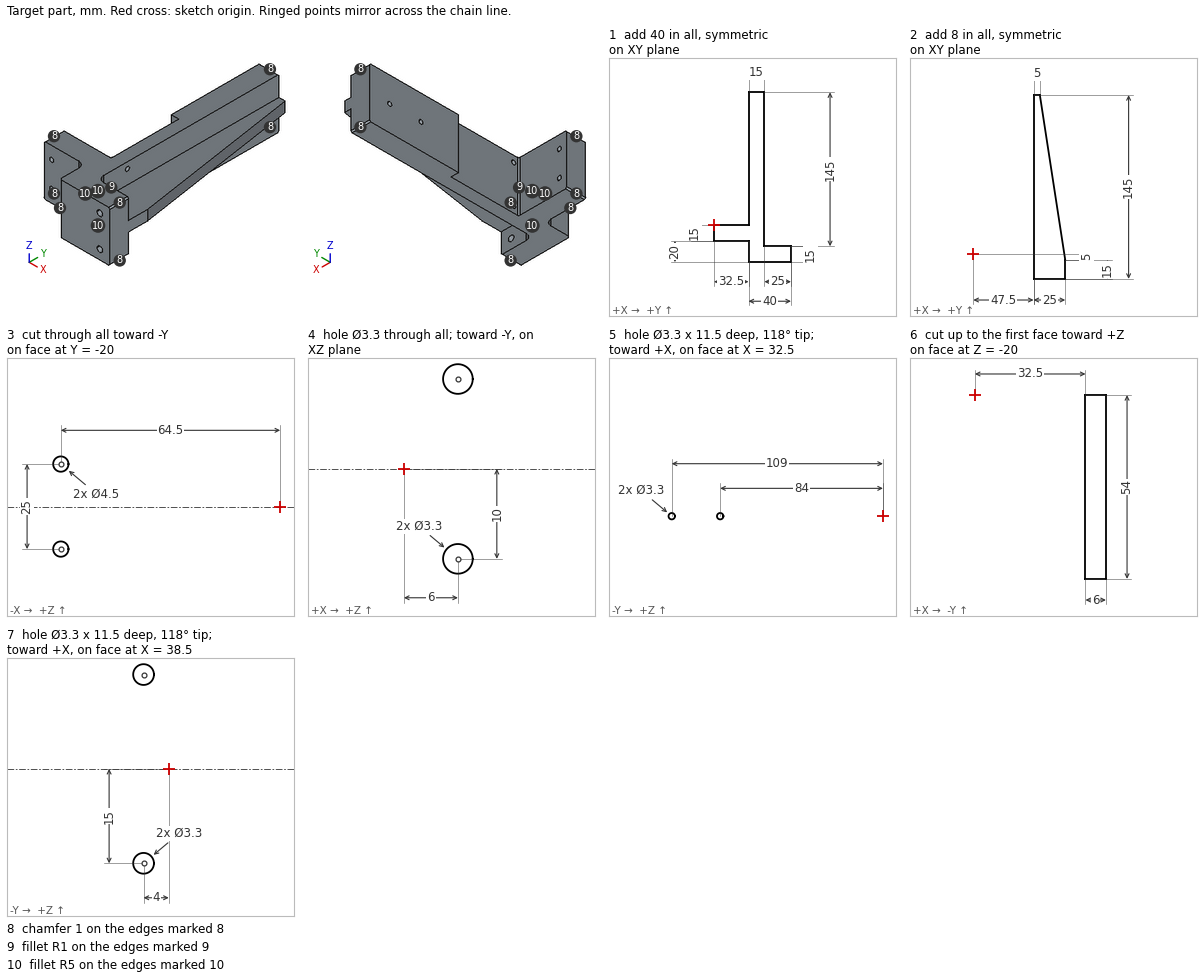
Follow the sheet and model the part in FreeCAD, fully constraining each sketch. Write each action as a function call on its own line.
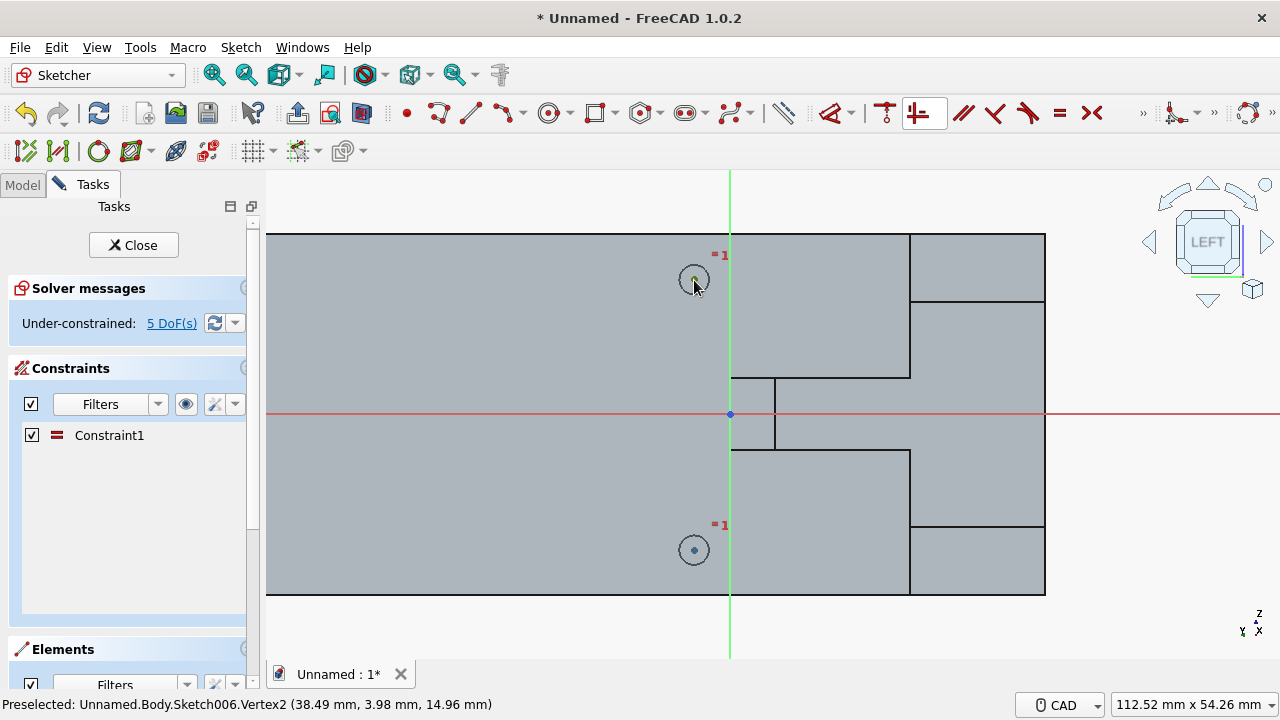
click(353, 414)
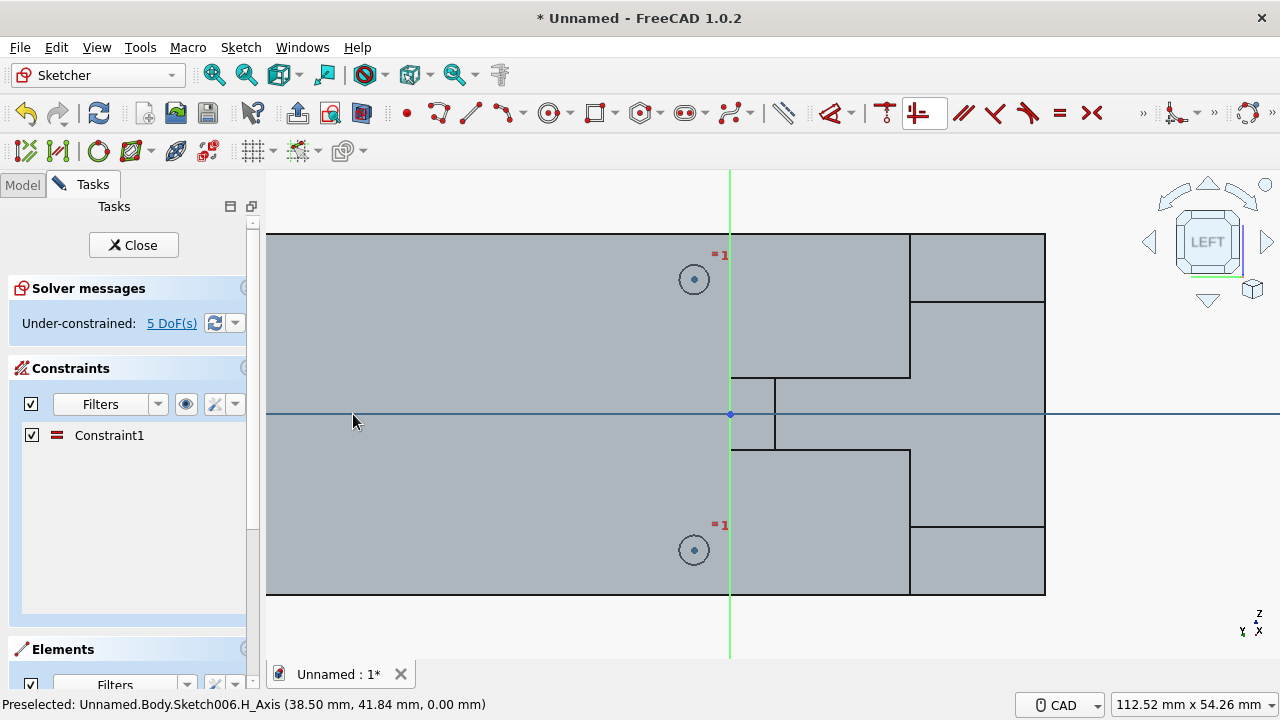
click(1092, 114)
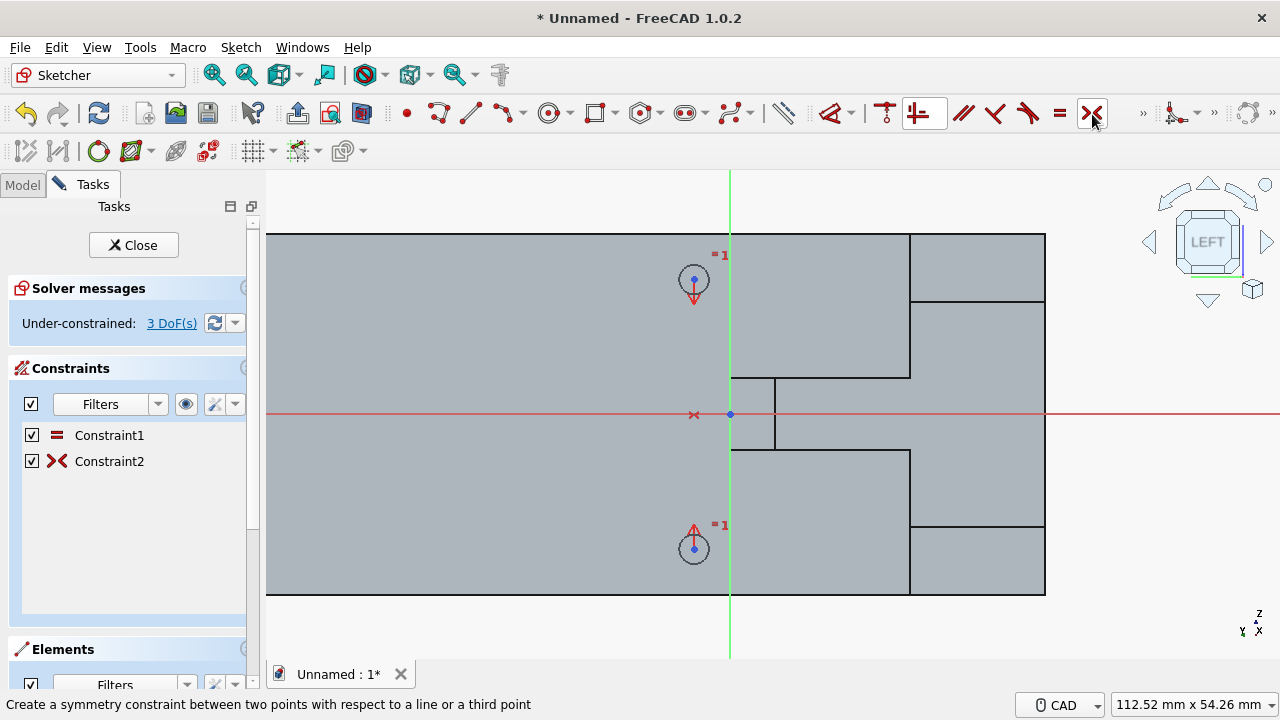
key(d)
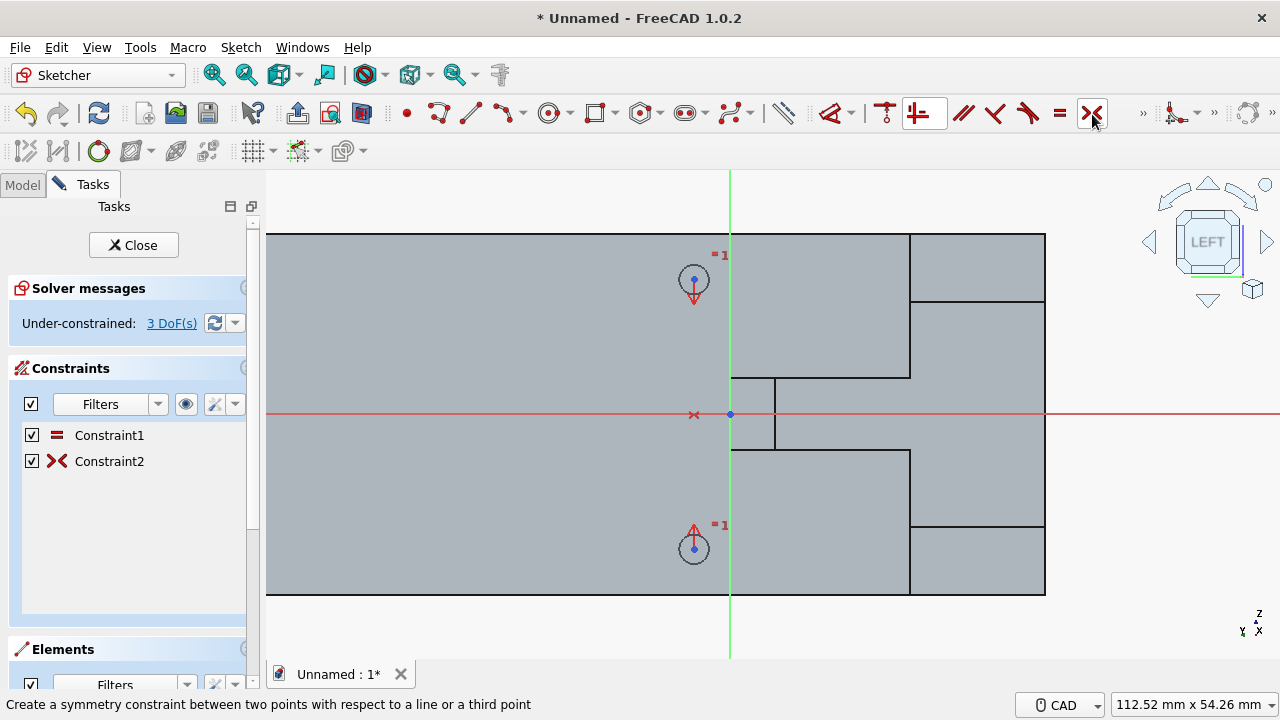
scroll(704, 539, up, 2)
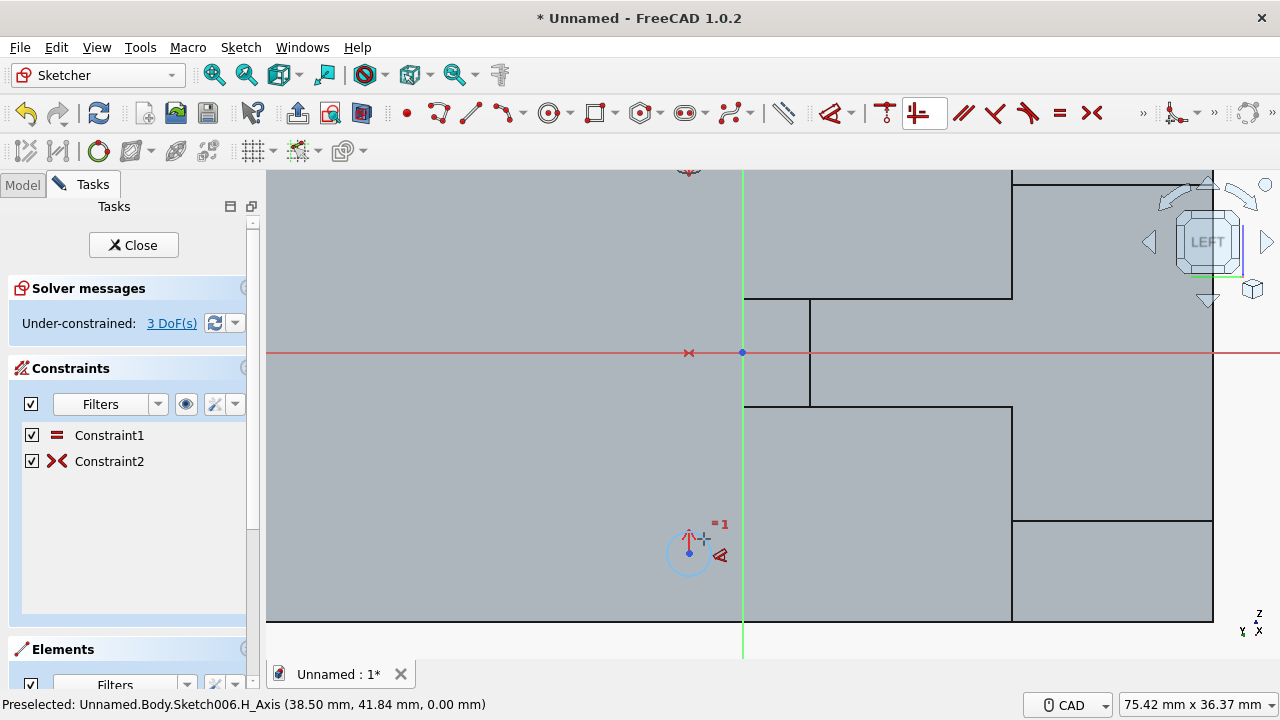
click(705, 538)
click(728, 515)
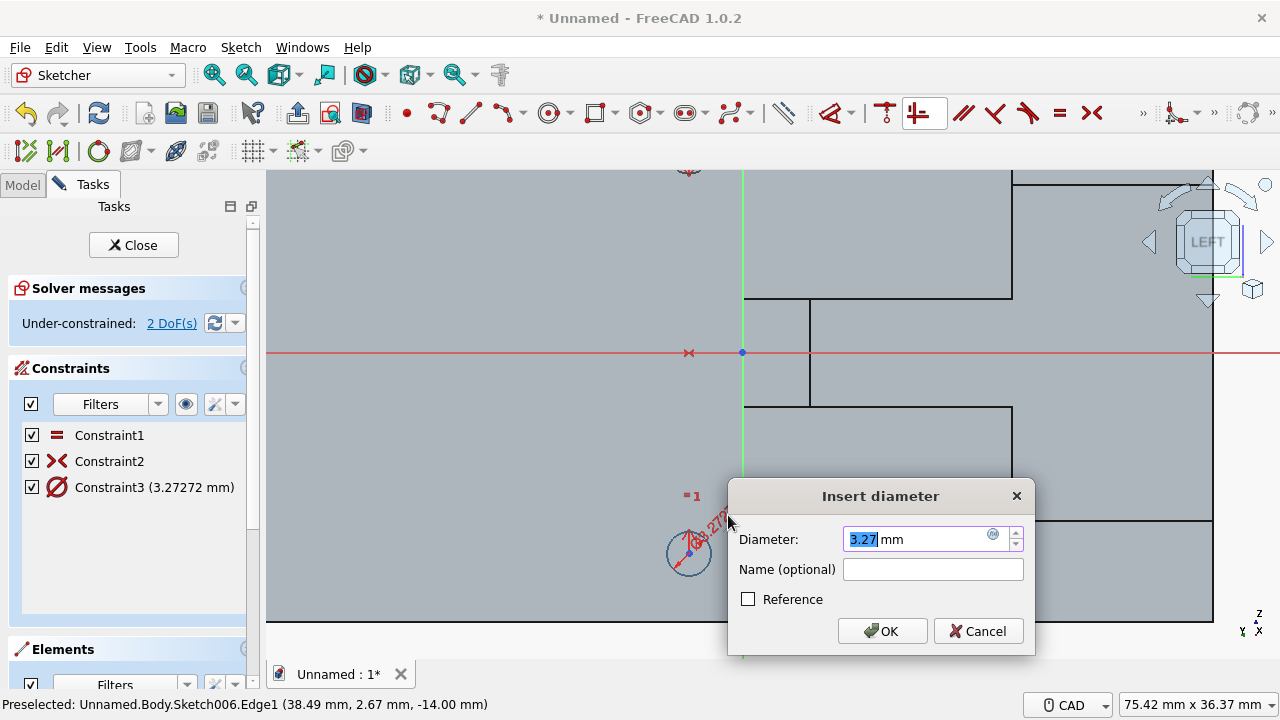
text(3.3)
key(Return)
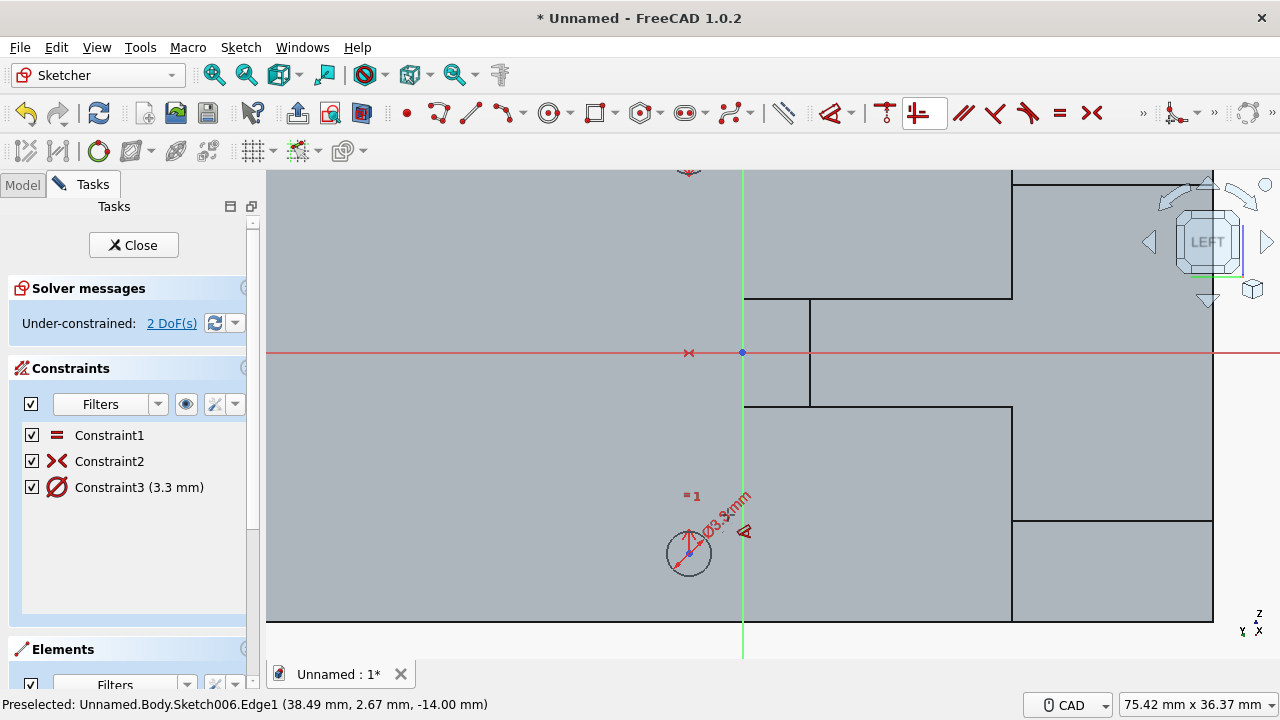
click(689, 554)
click(716, 588)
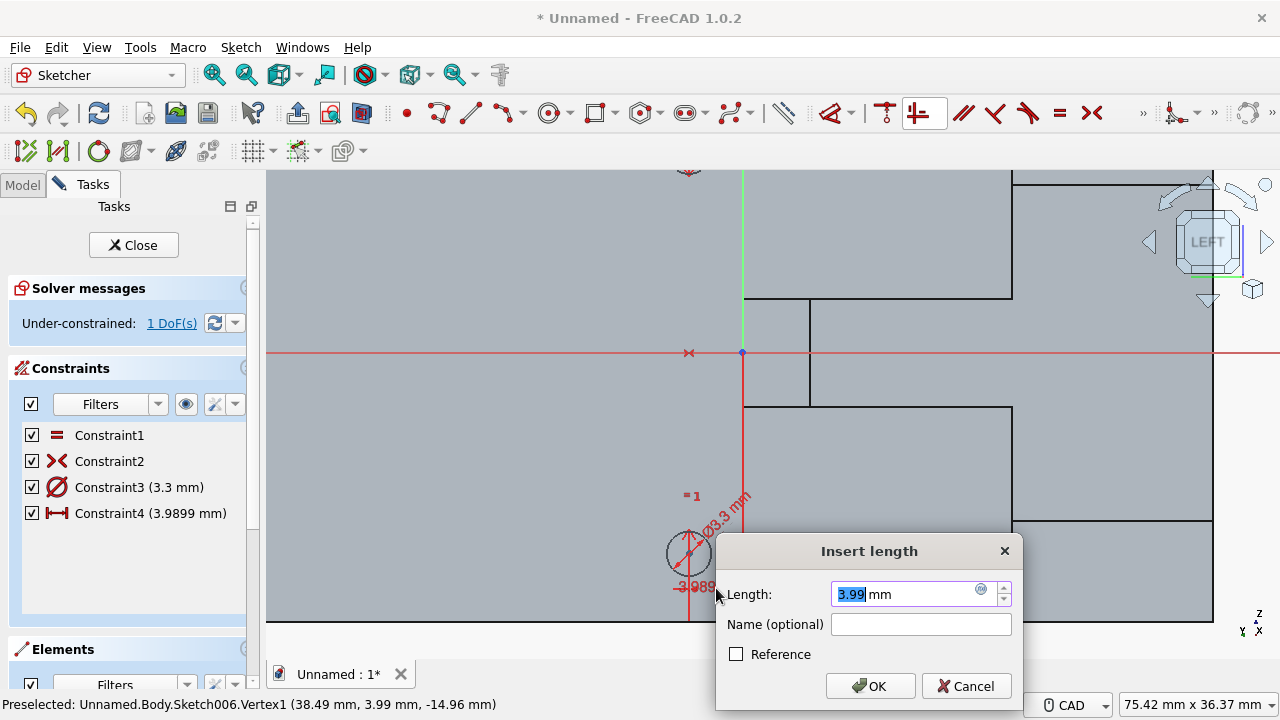
text(4)
key(Return)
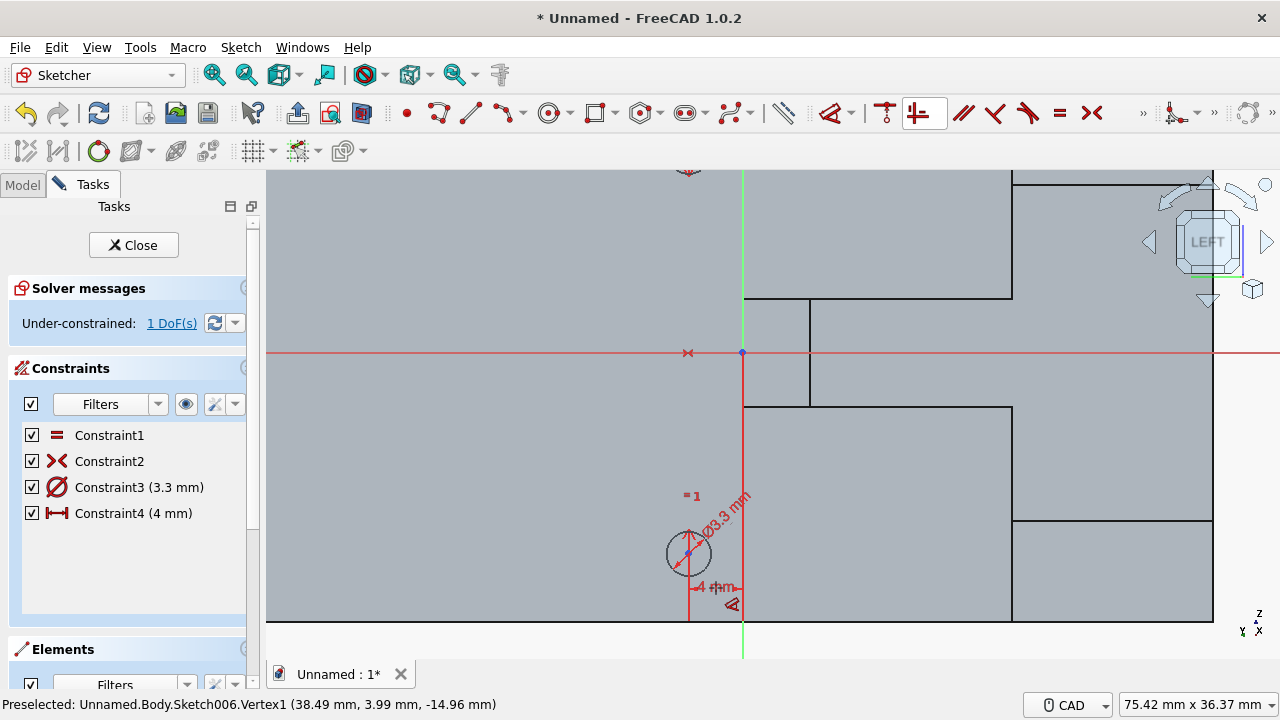
click(689, 554)
click(777, 453)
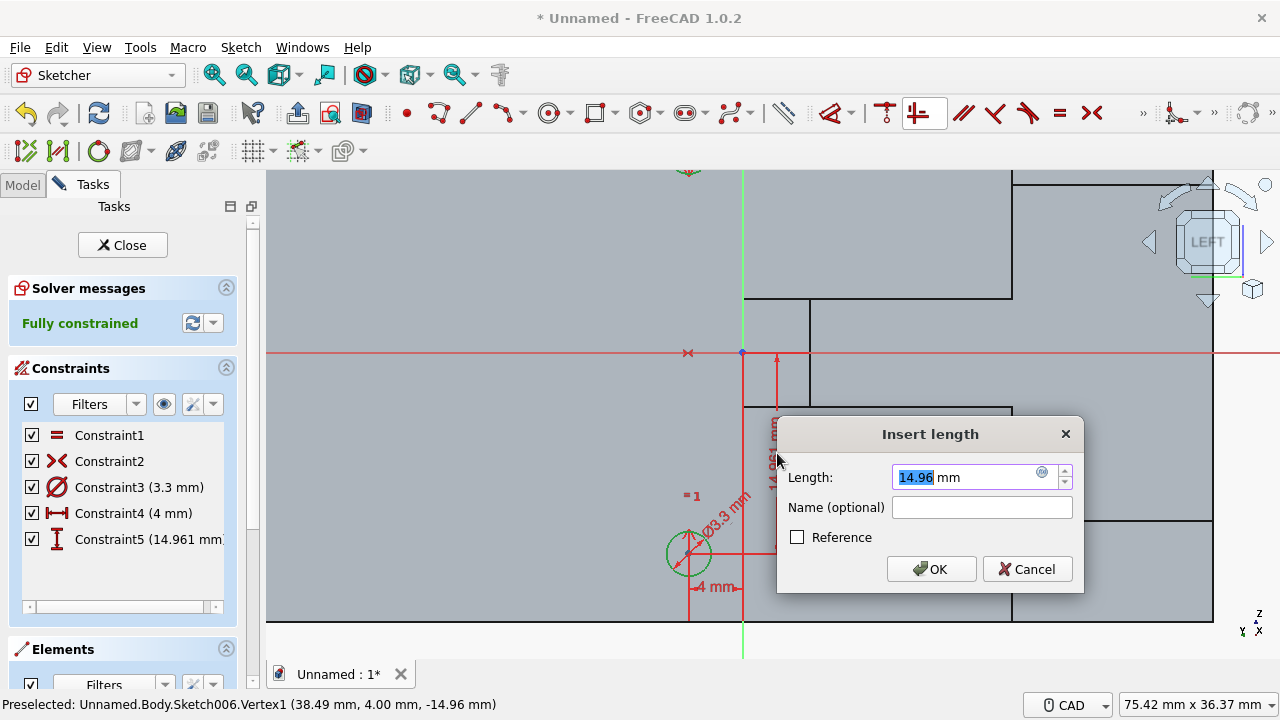
text(15)
key(Return)
key(Escape)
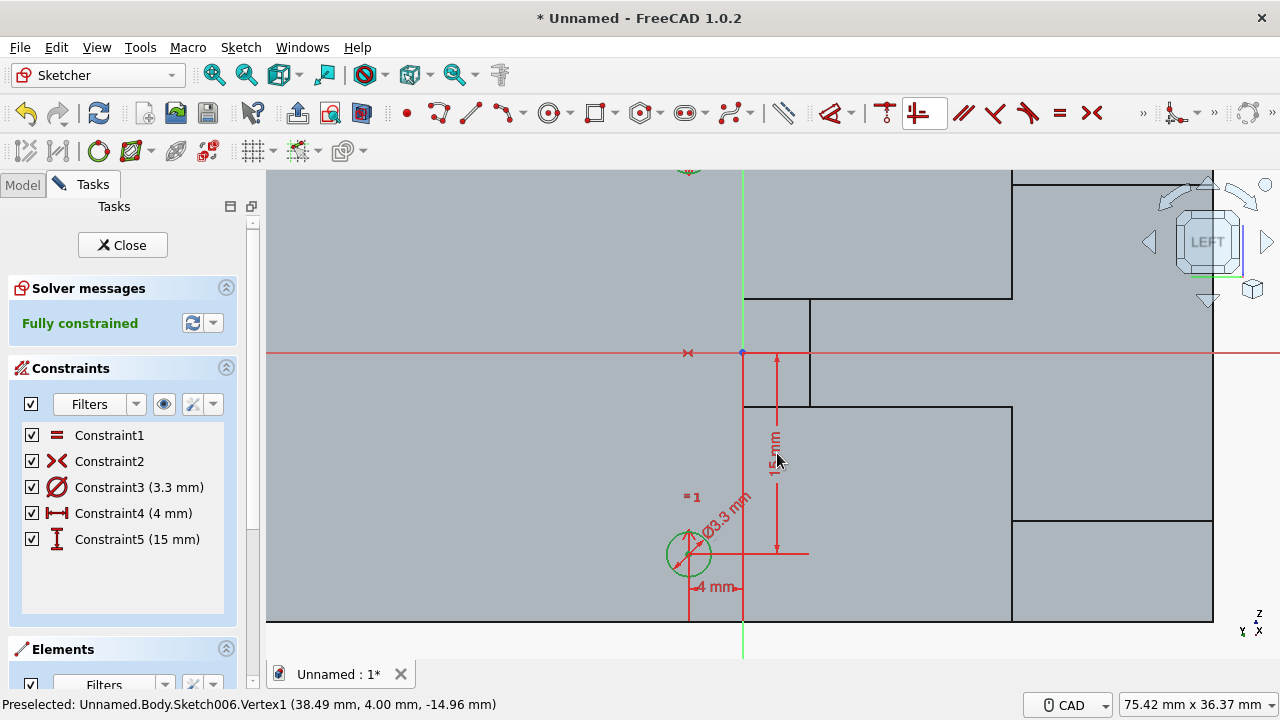
click(123, 245)